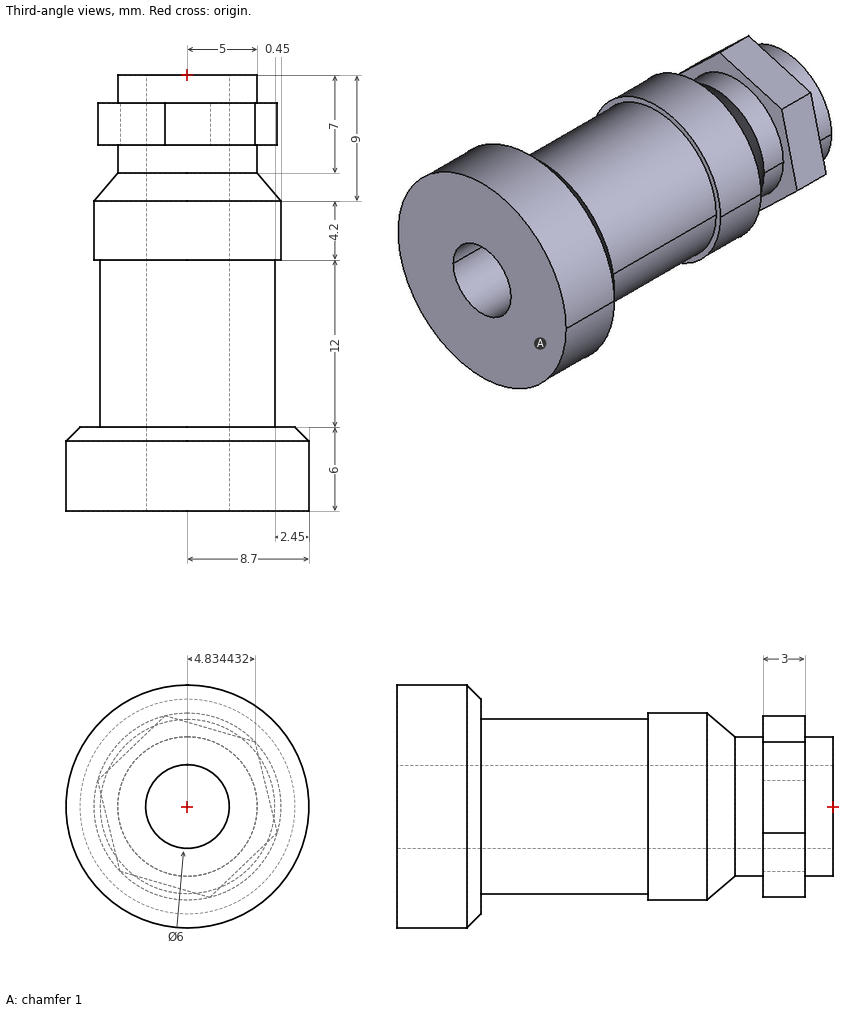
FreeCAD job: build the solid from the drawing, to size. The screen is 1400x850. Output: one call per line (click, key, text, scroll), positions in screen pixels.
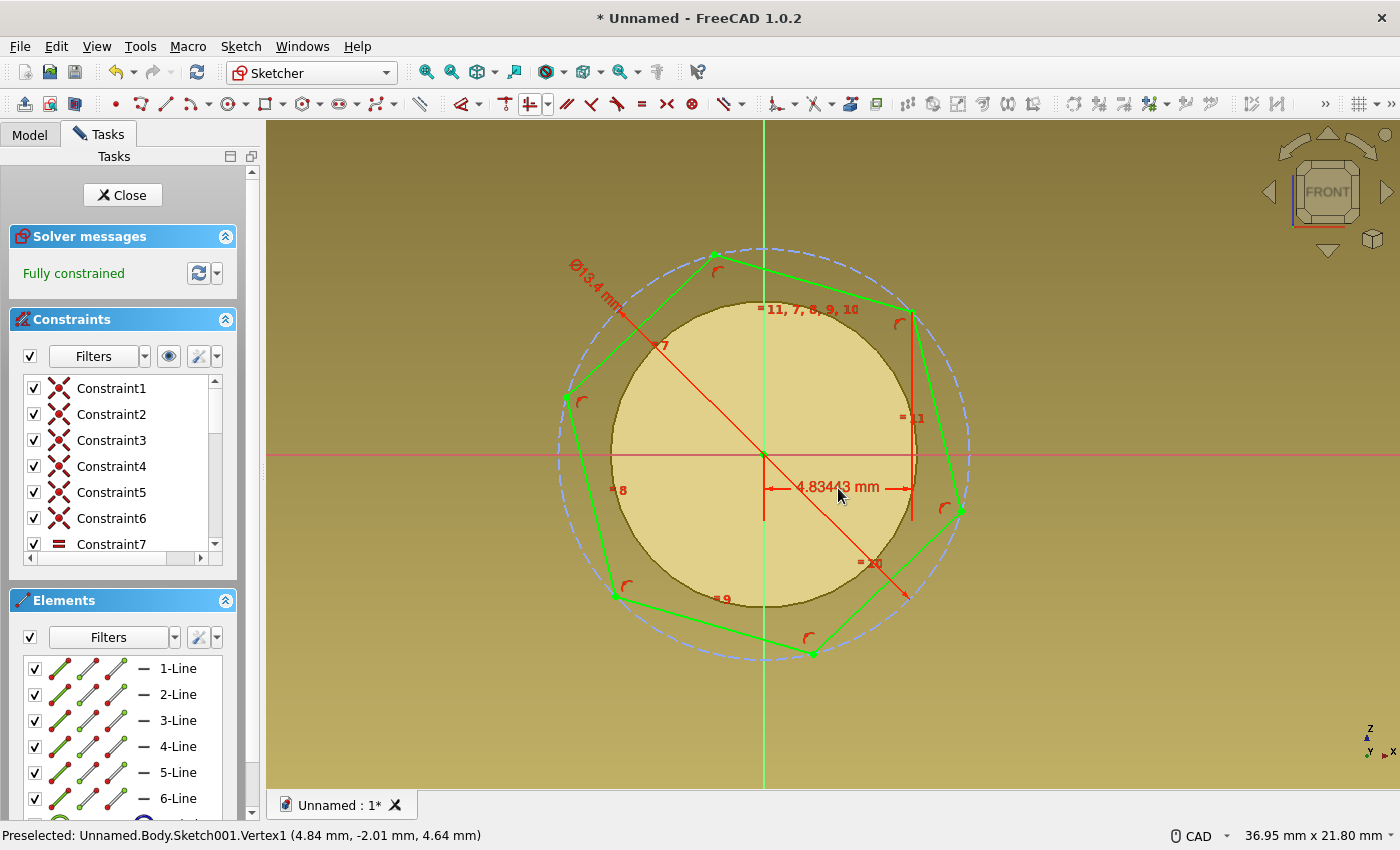
click(123, 195)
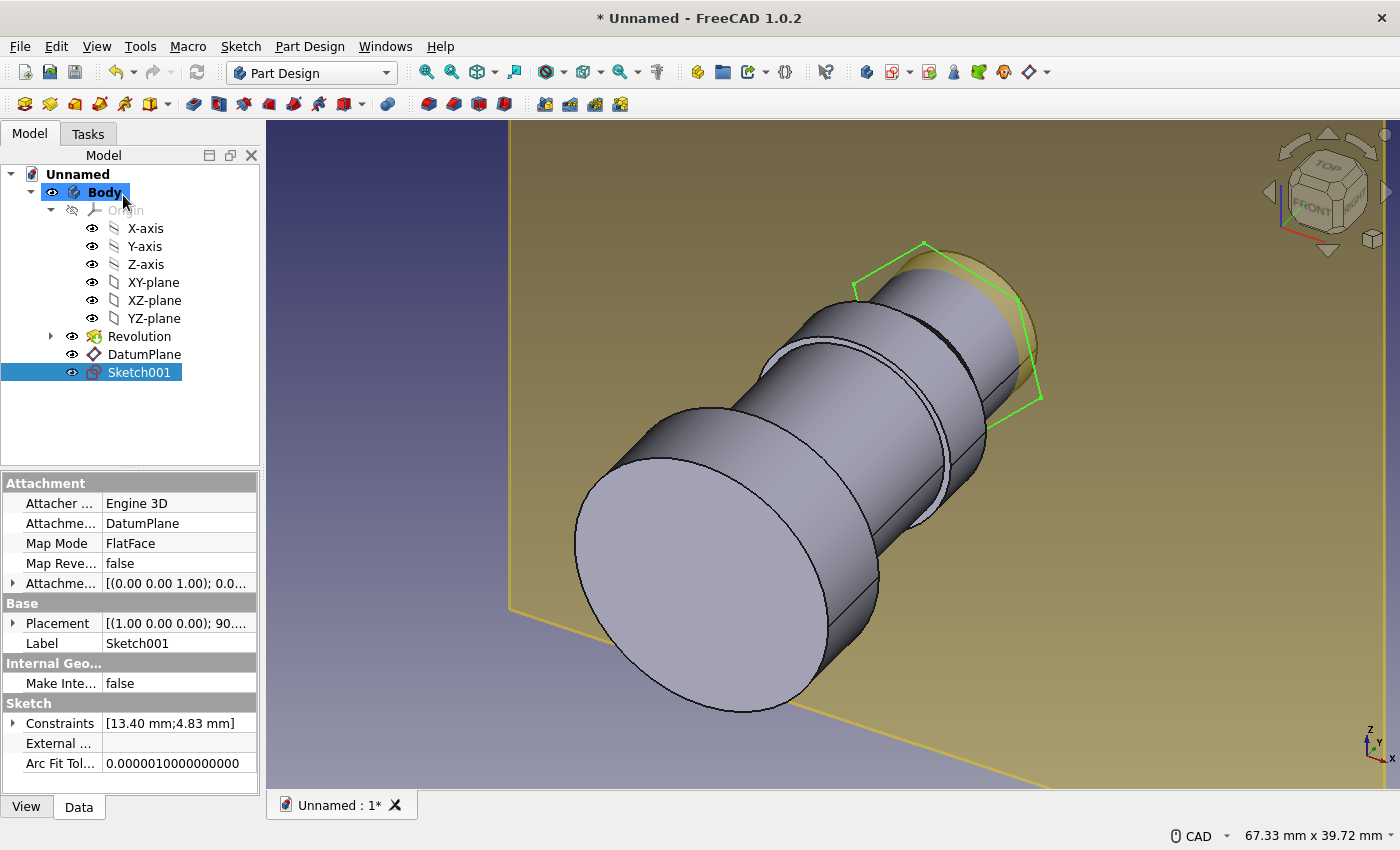
click(25, 104)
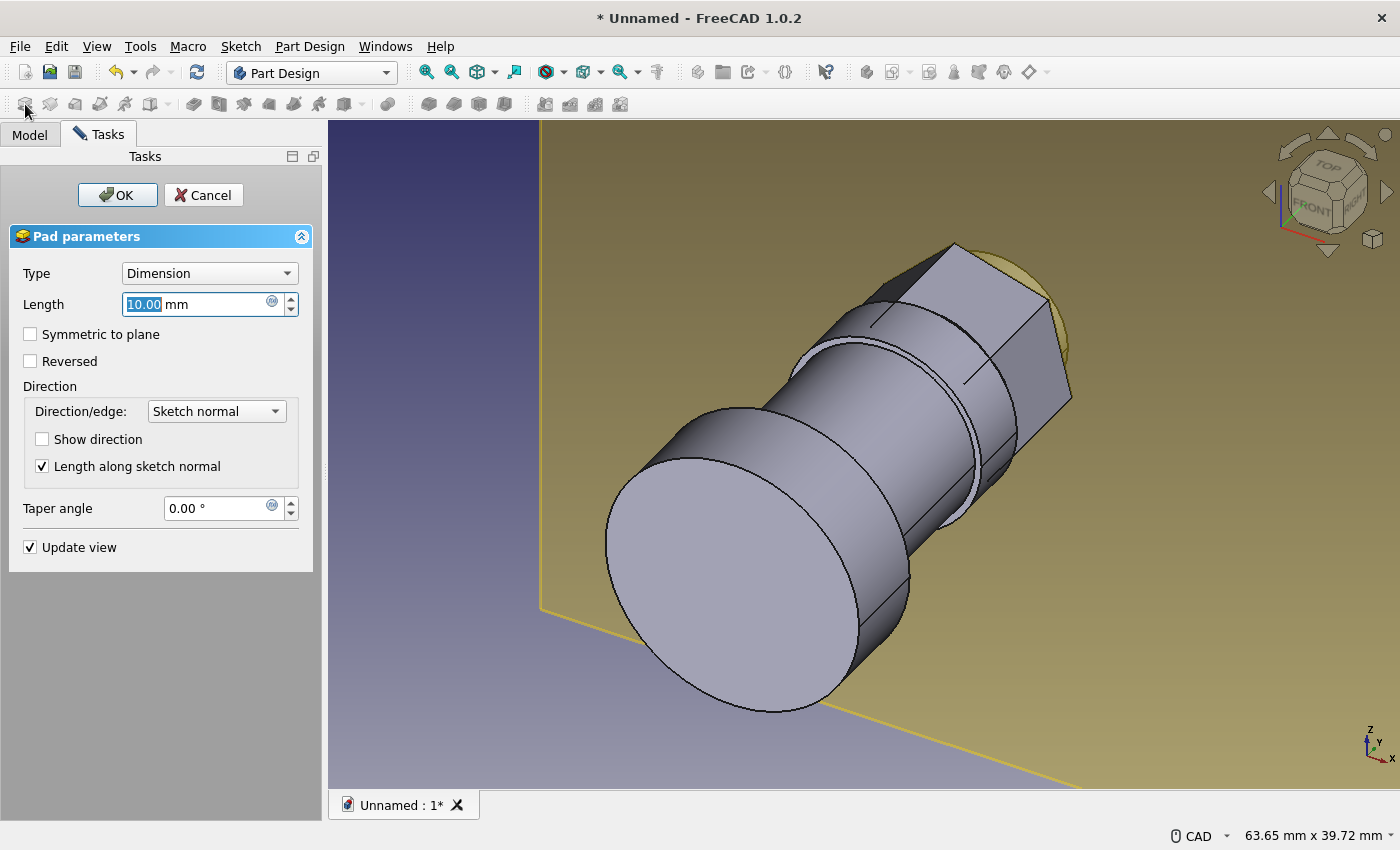
text(3)
key(Tab)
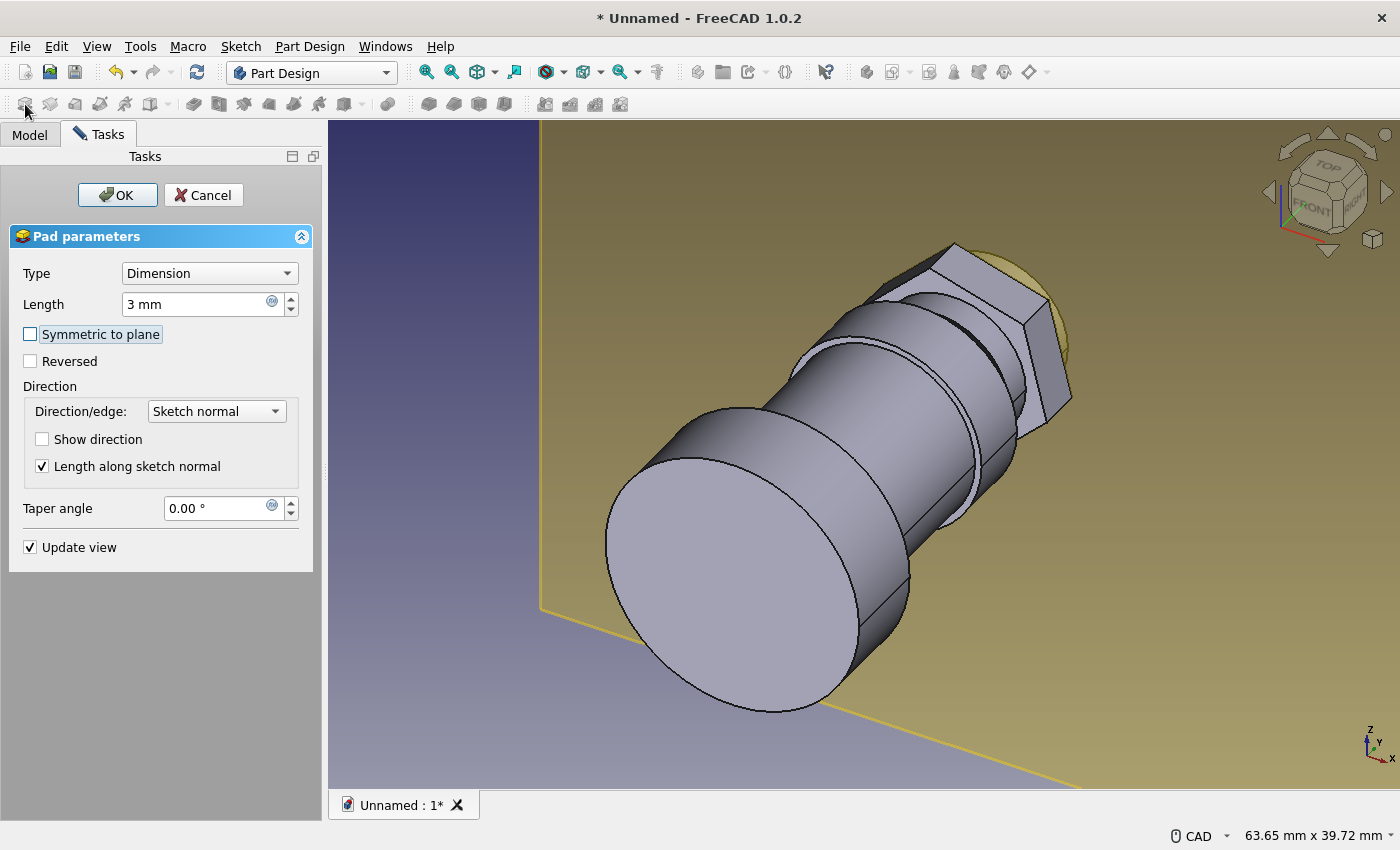
click(118, 195)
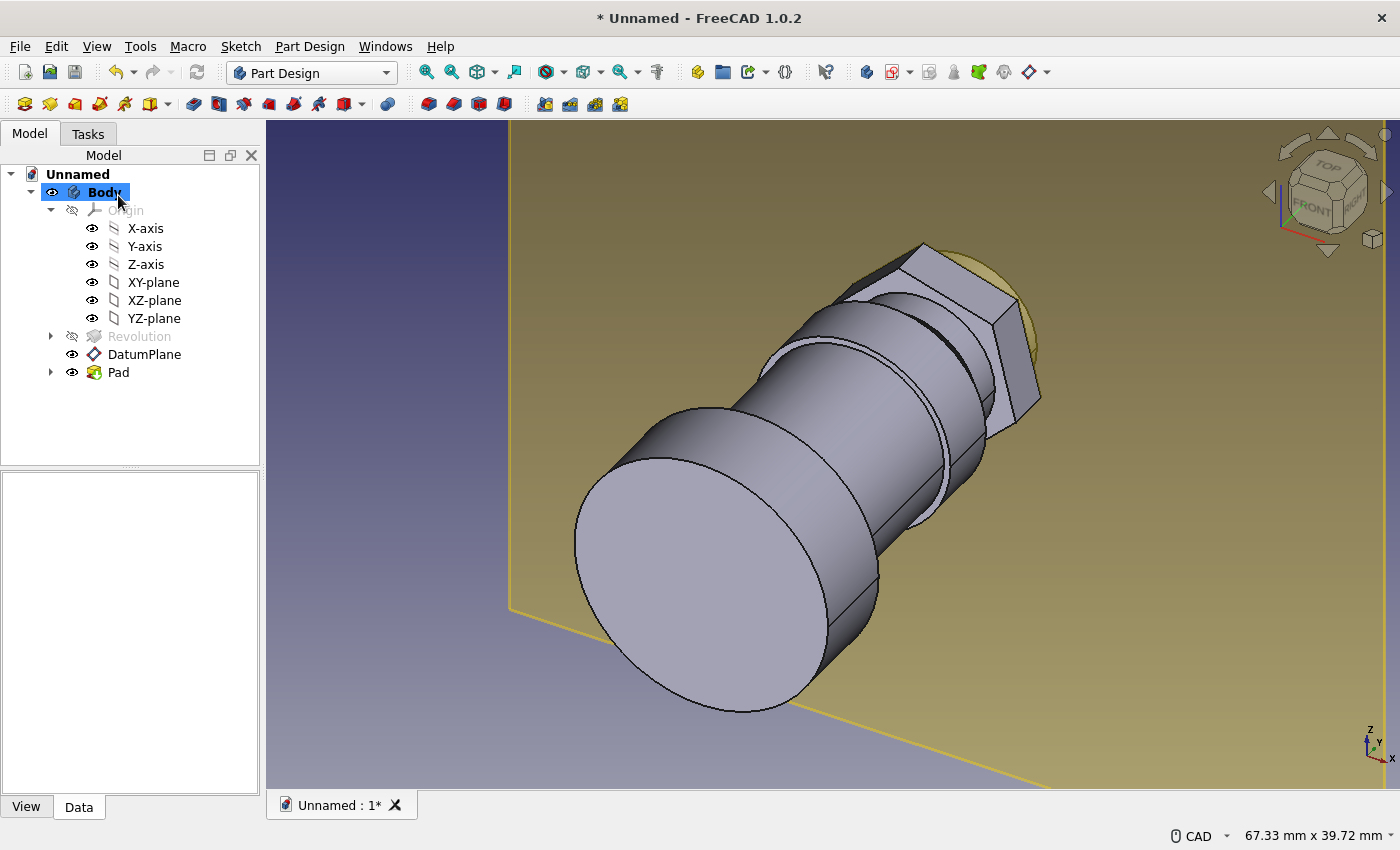
click(117, 354)
key(space)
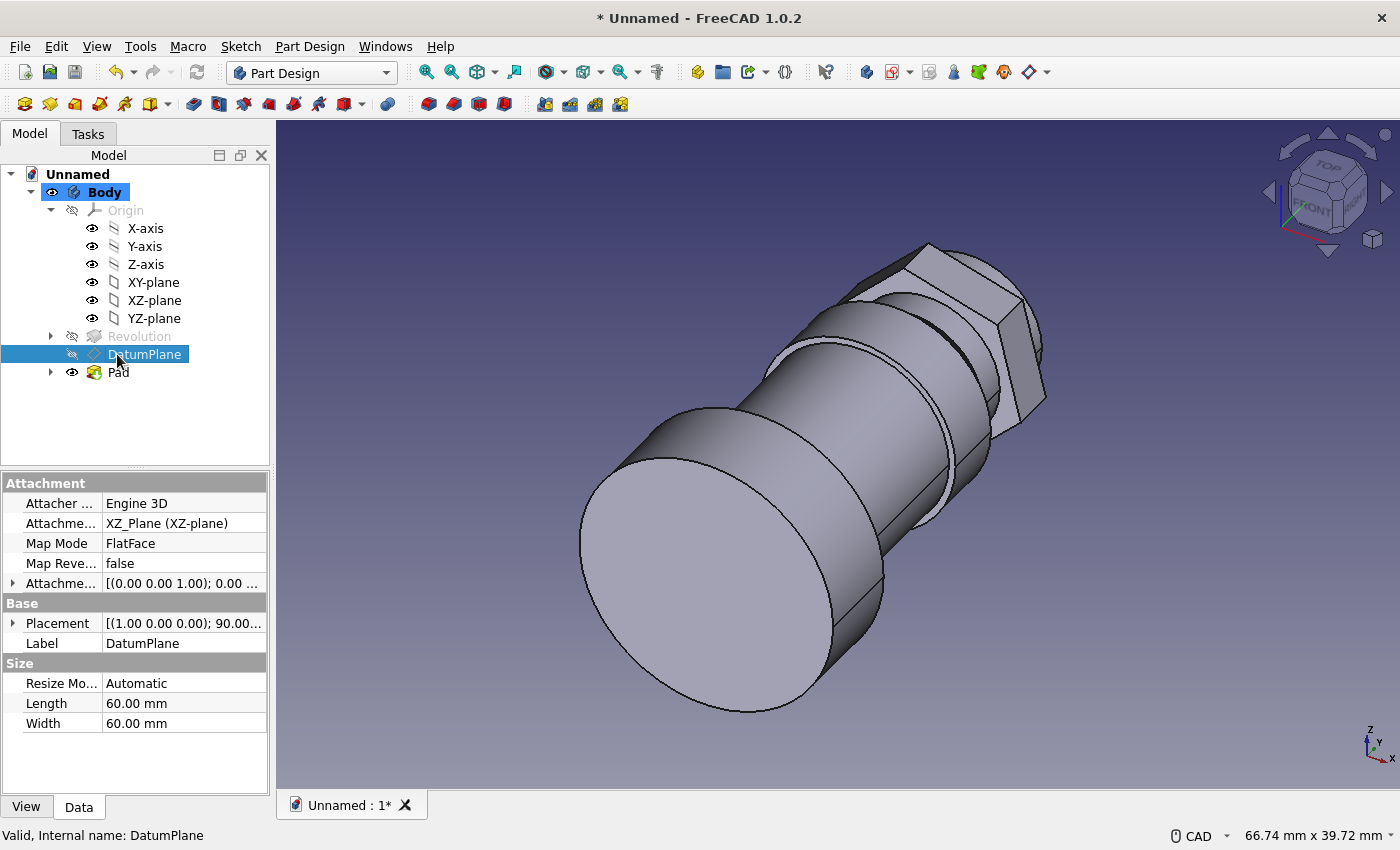
key(4)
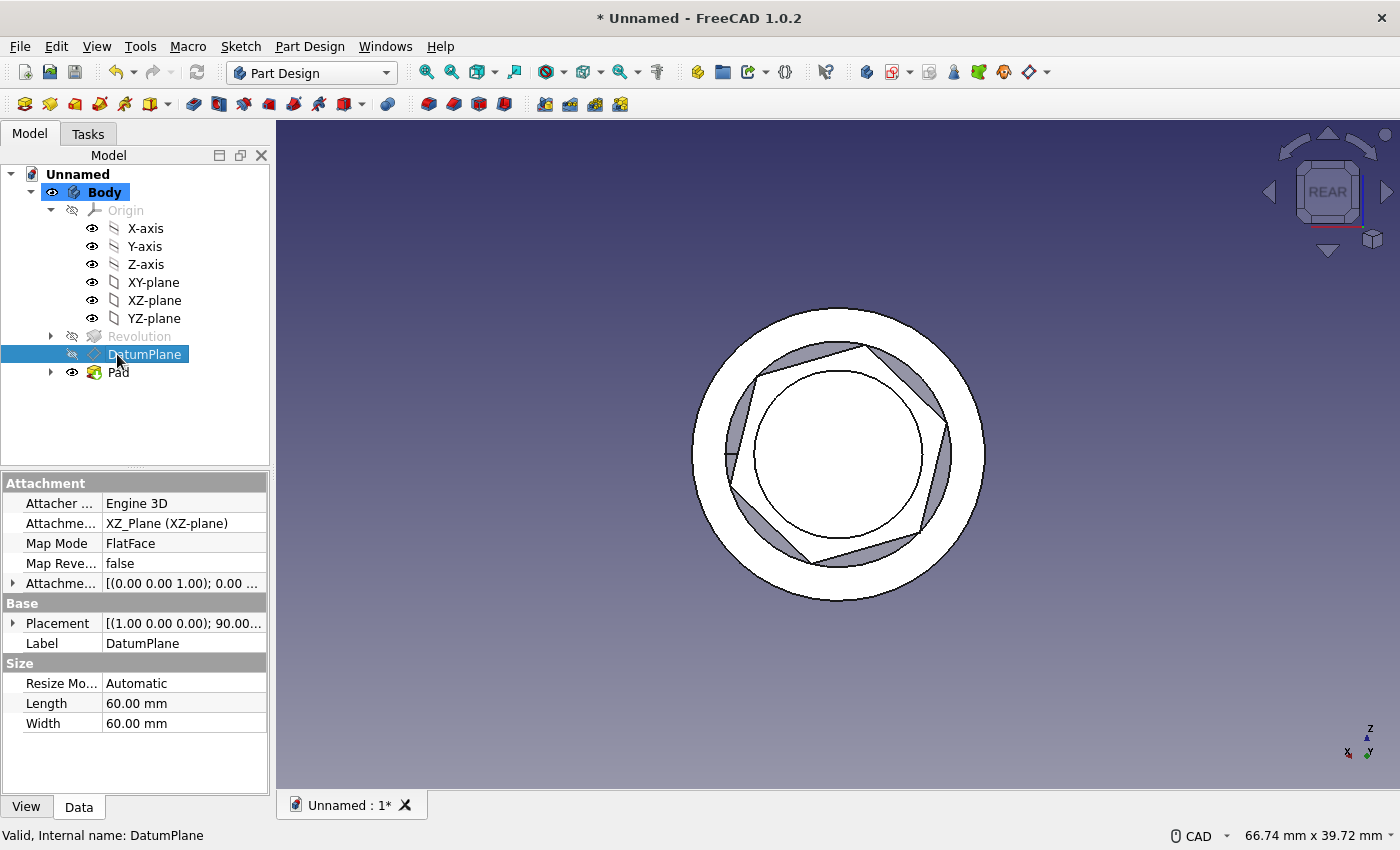
click(427, 72)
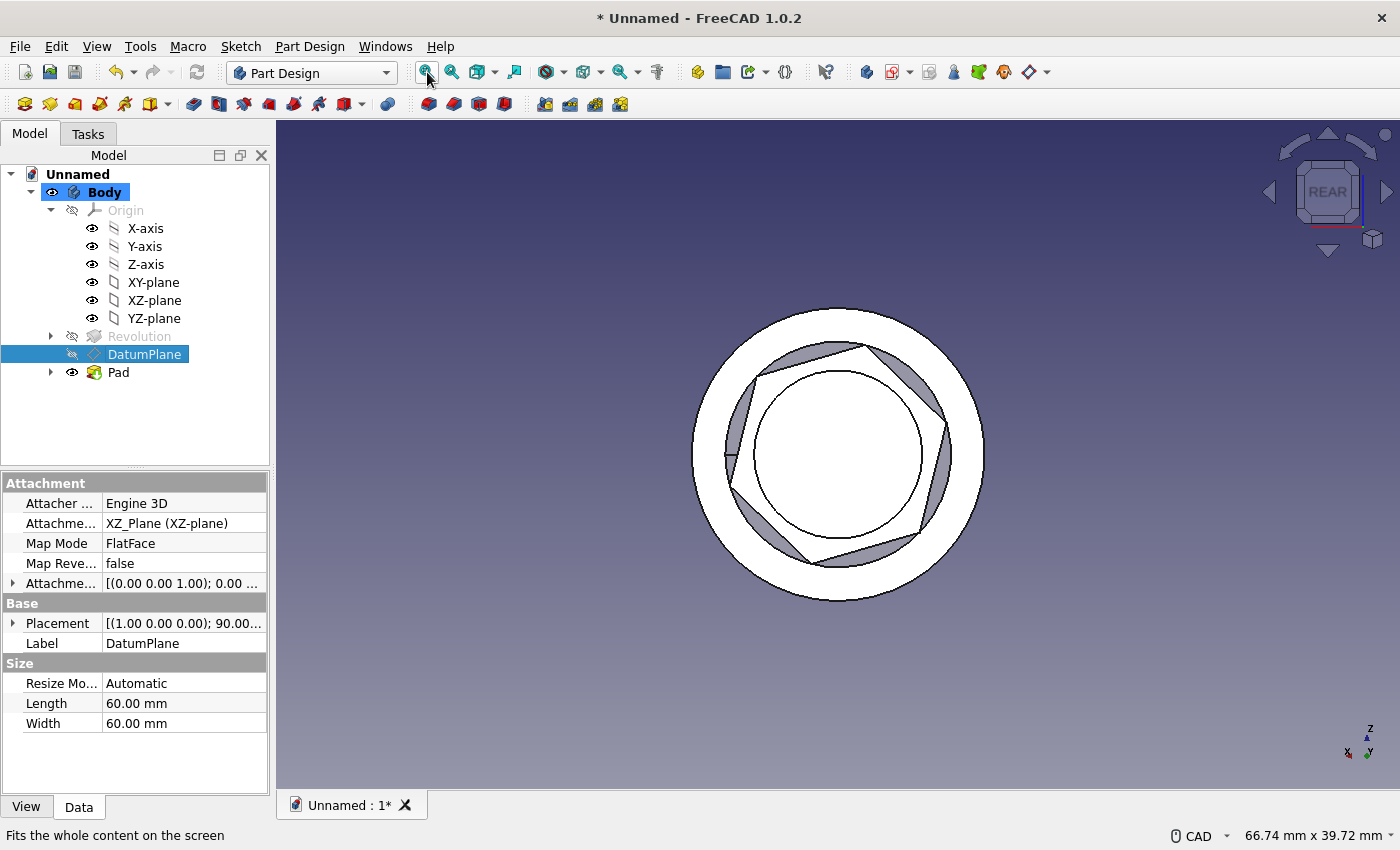
click(838, 454)